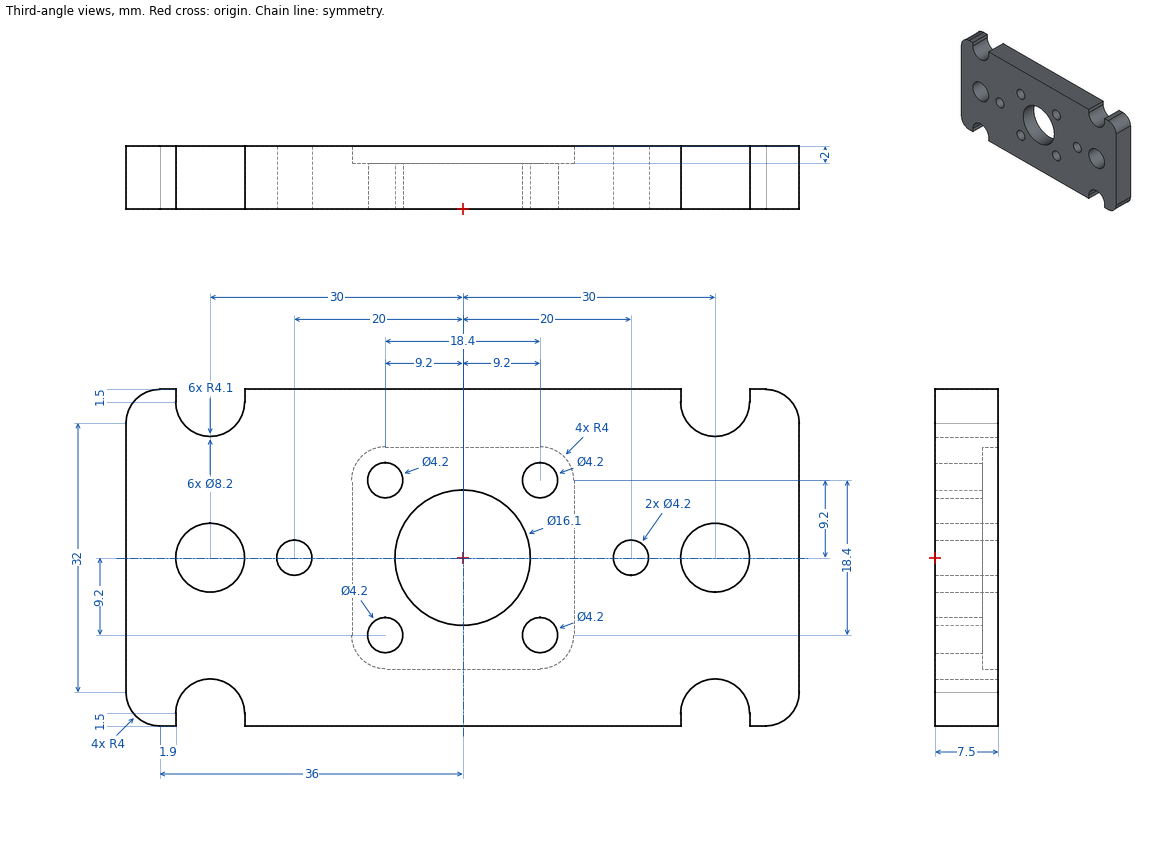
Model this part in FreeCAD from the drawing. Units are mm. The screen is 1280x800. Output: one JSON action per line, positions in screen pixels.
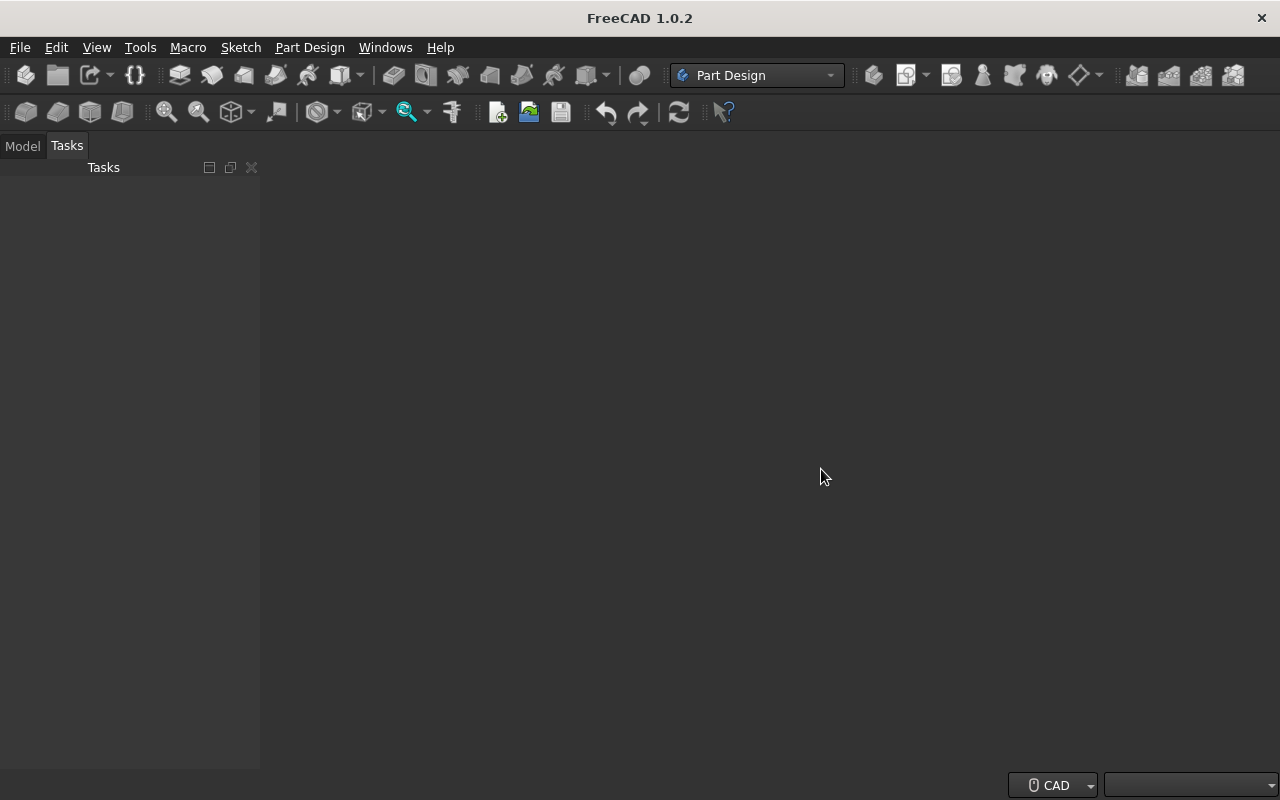
{"action": "left_click", "coordinate": [498, 112]}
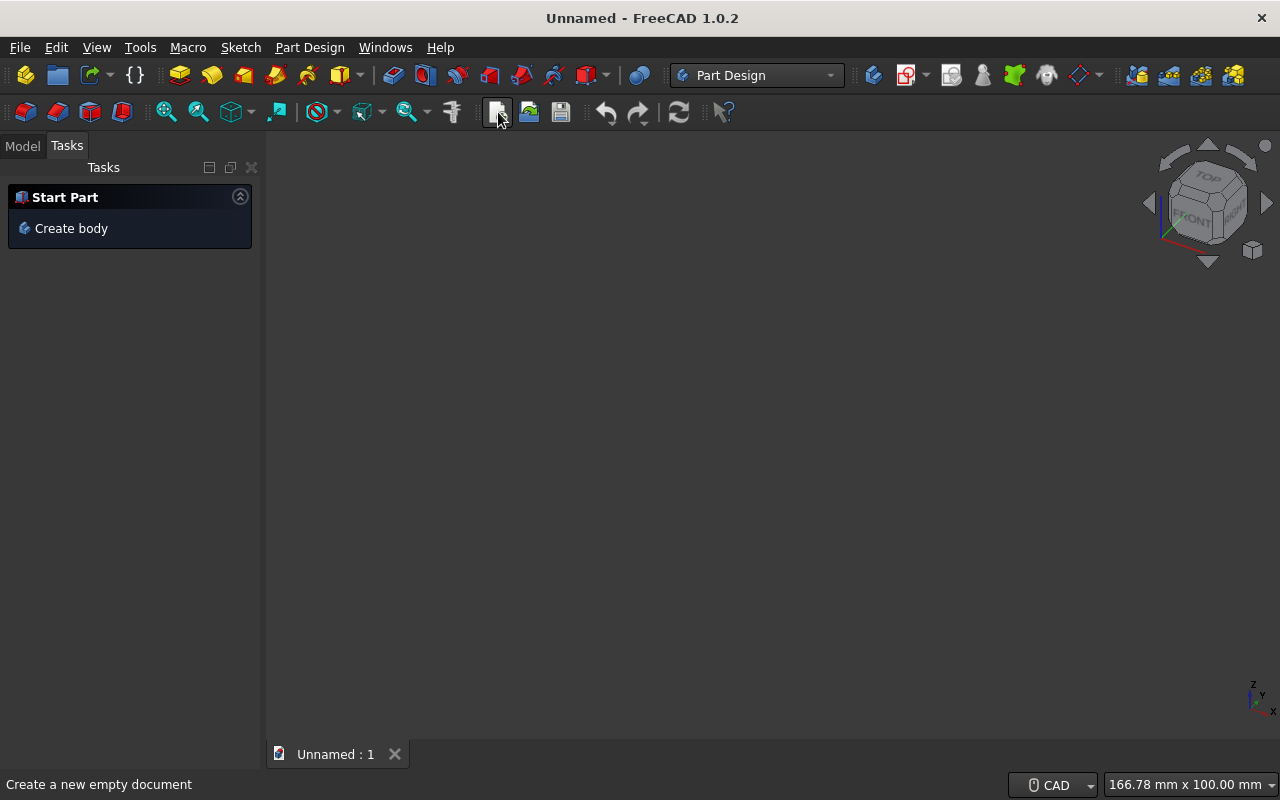
{"action": "left_click", "coordinate": [906, 76]}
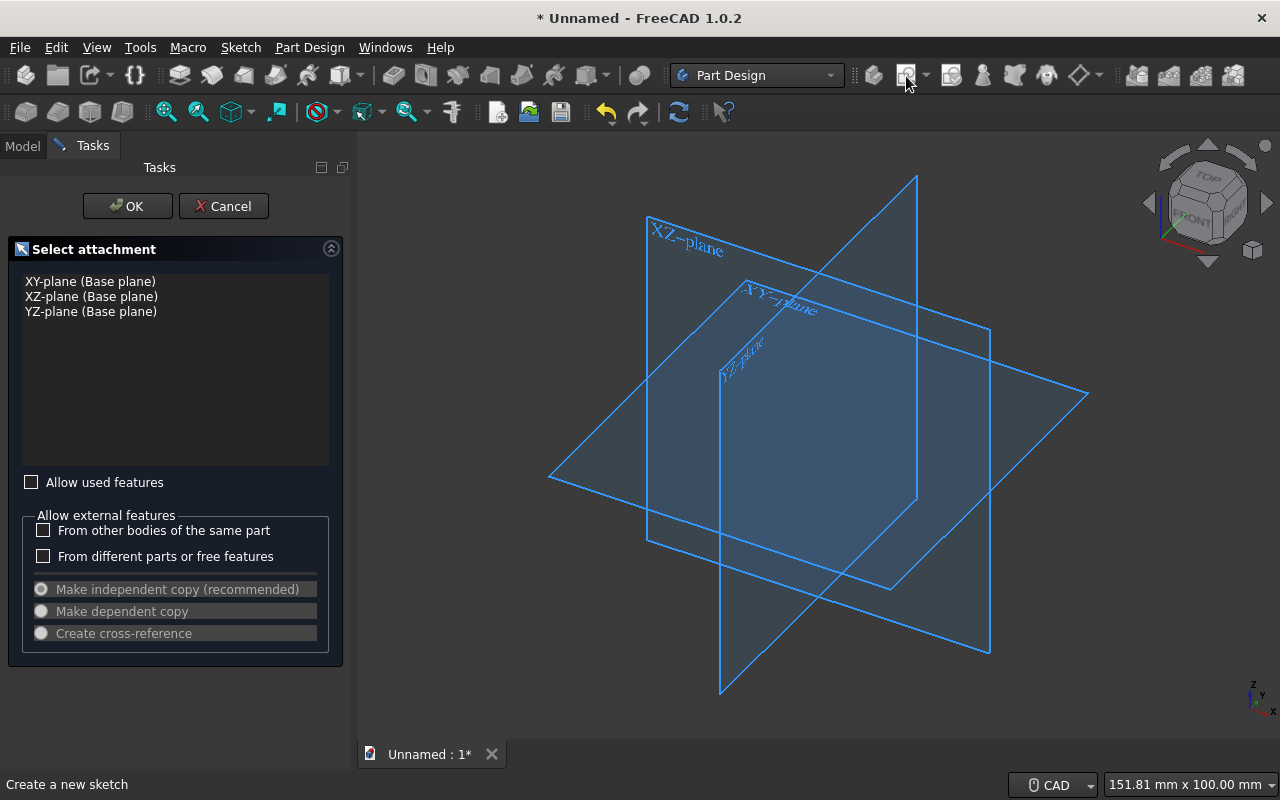
{"action": "left_click", "coordinate": [82, 296]}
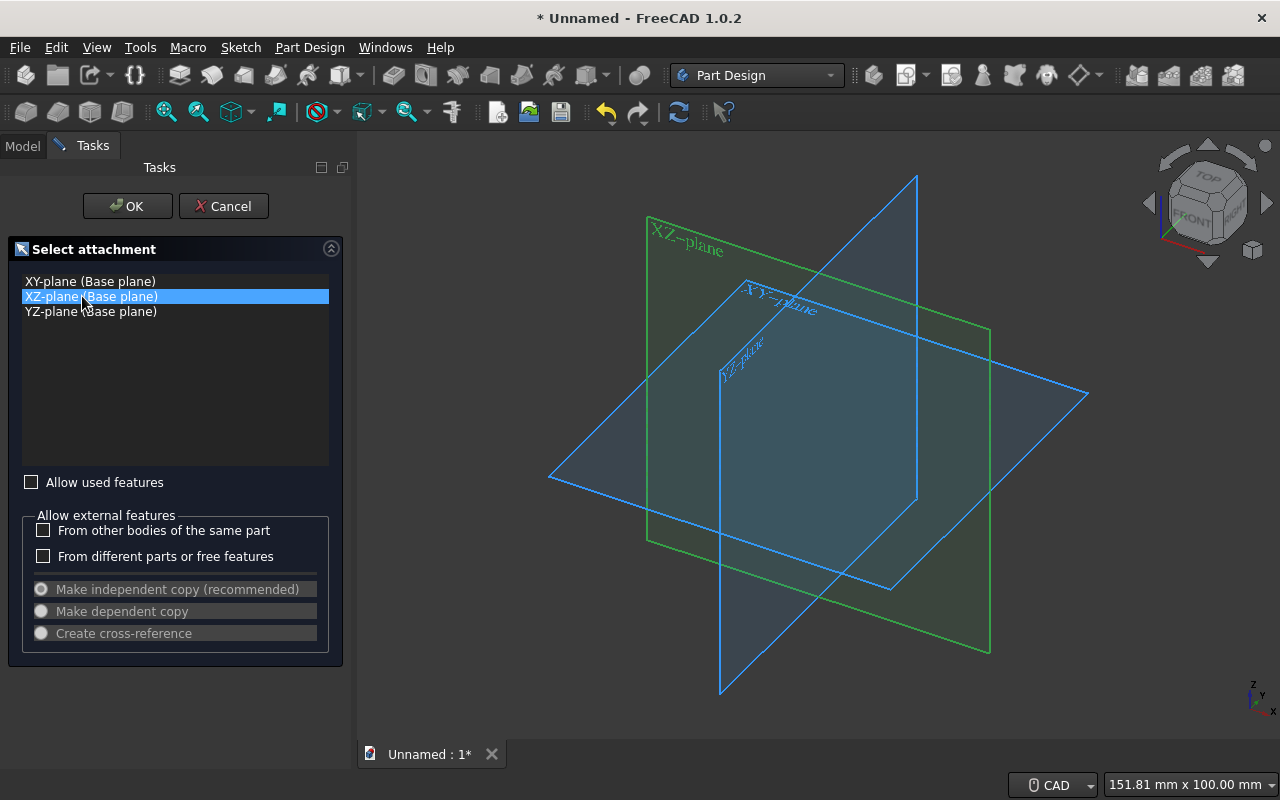
{"action": "left_click", "coordinate": [128, 206]}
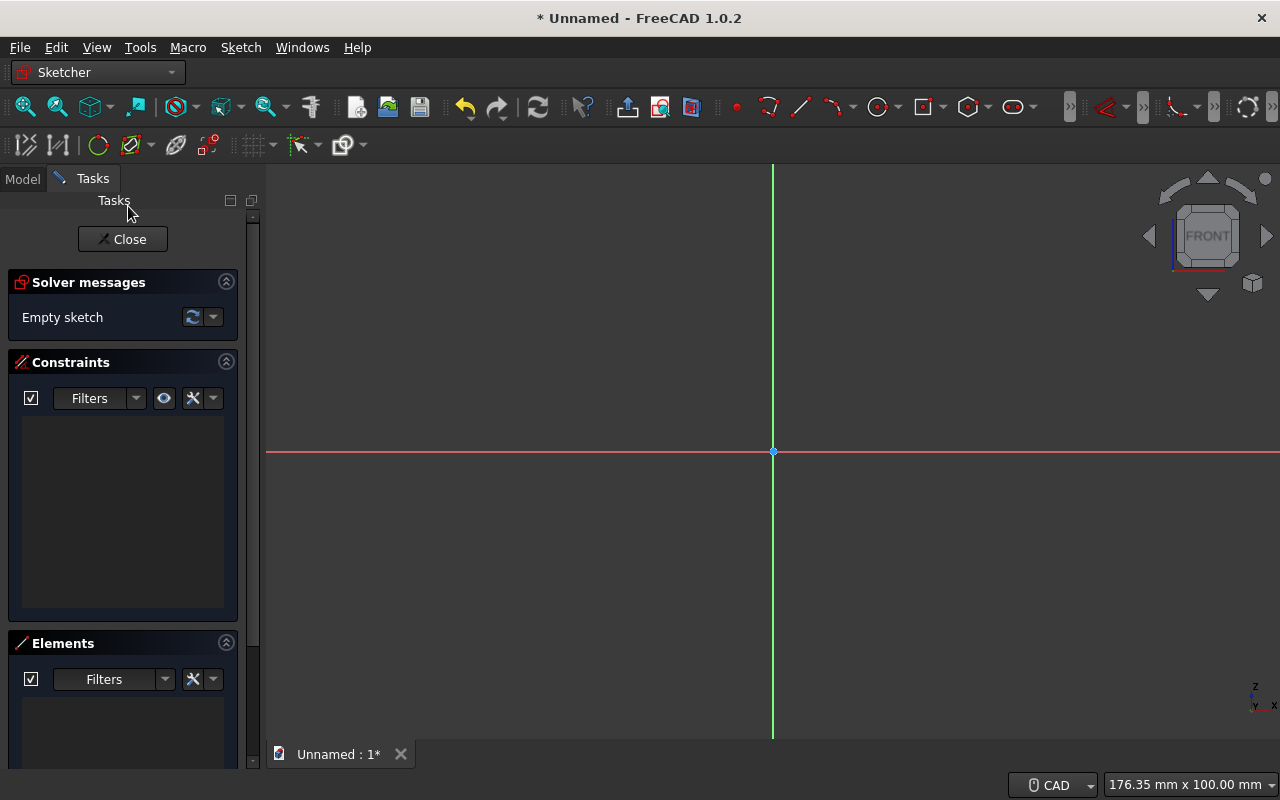
{"action": "left_click", "coordinate": [770, 108]}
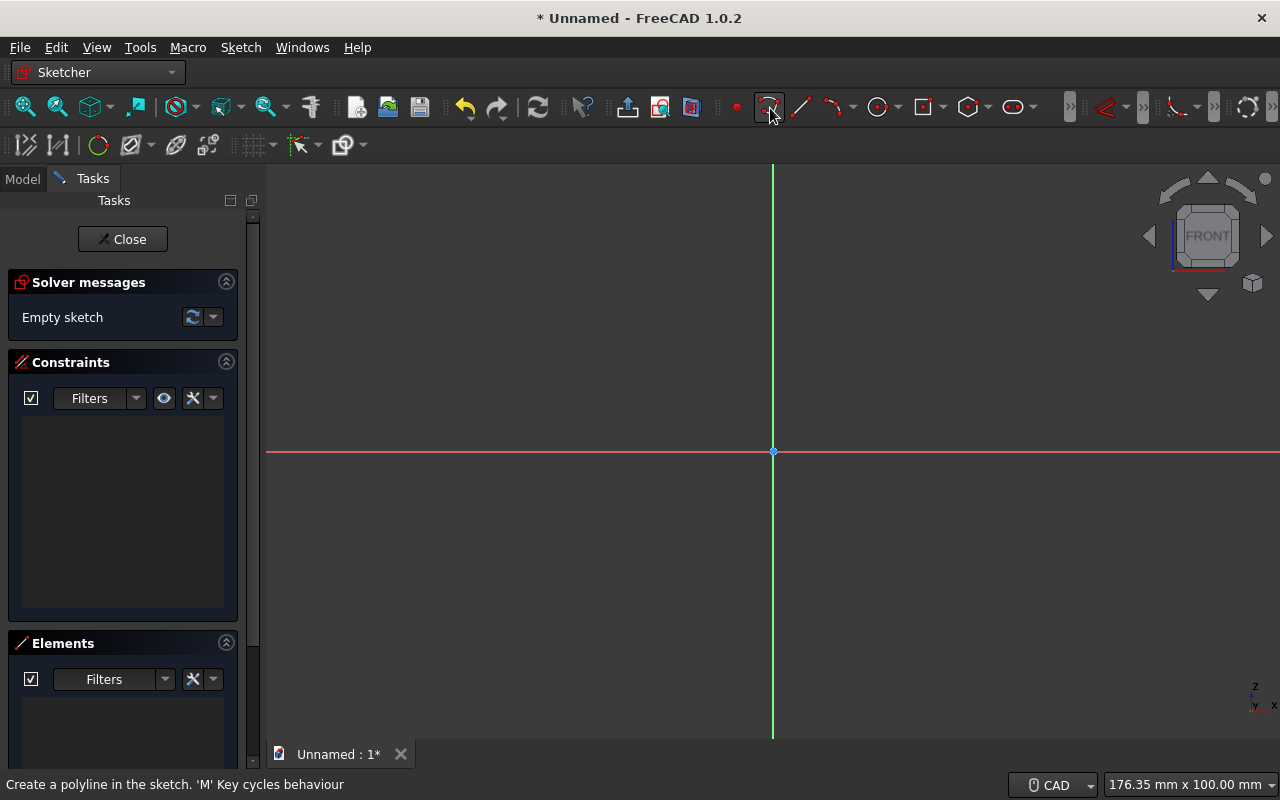
{"action": "left_click", "coordinate": [577, 558]}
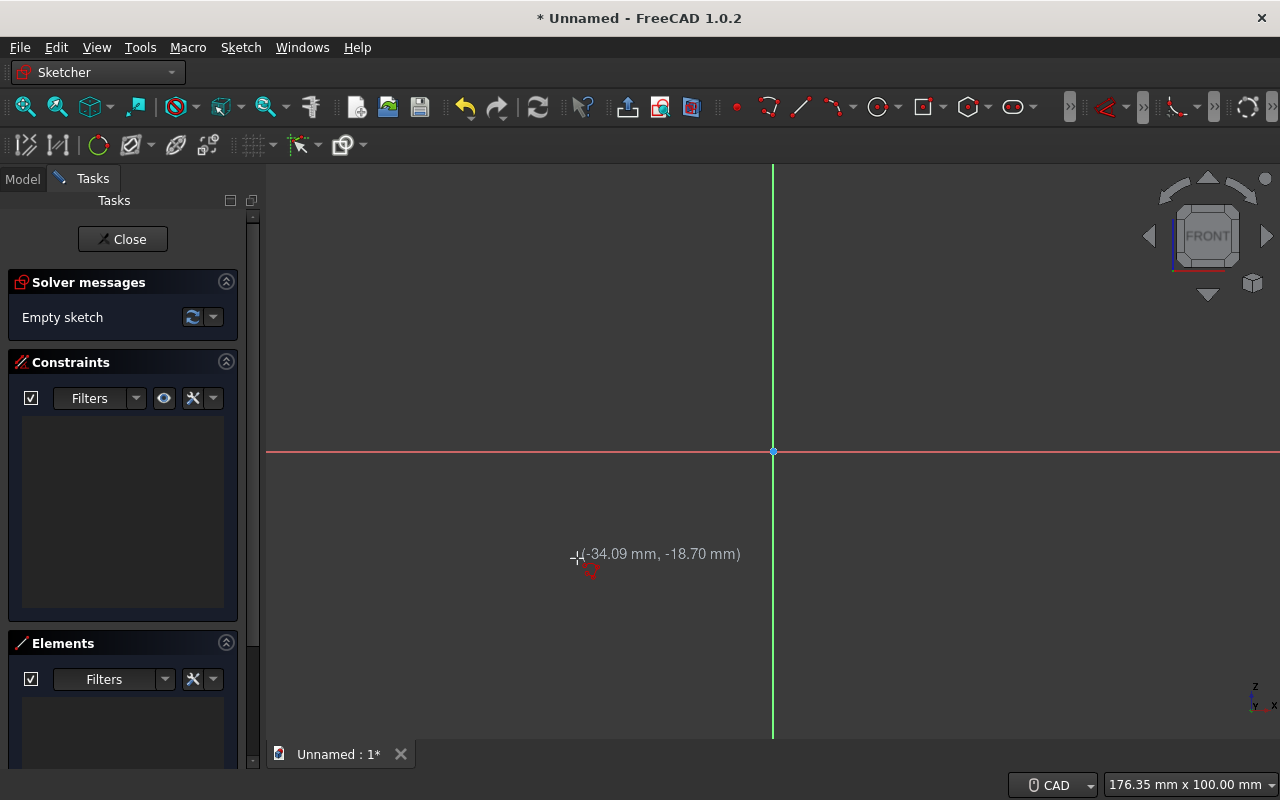
{"action": "scroll", "coordinate": [577, 566], "scroll_direction": "up", "scroll_amount": 4}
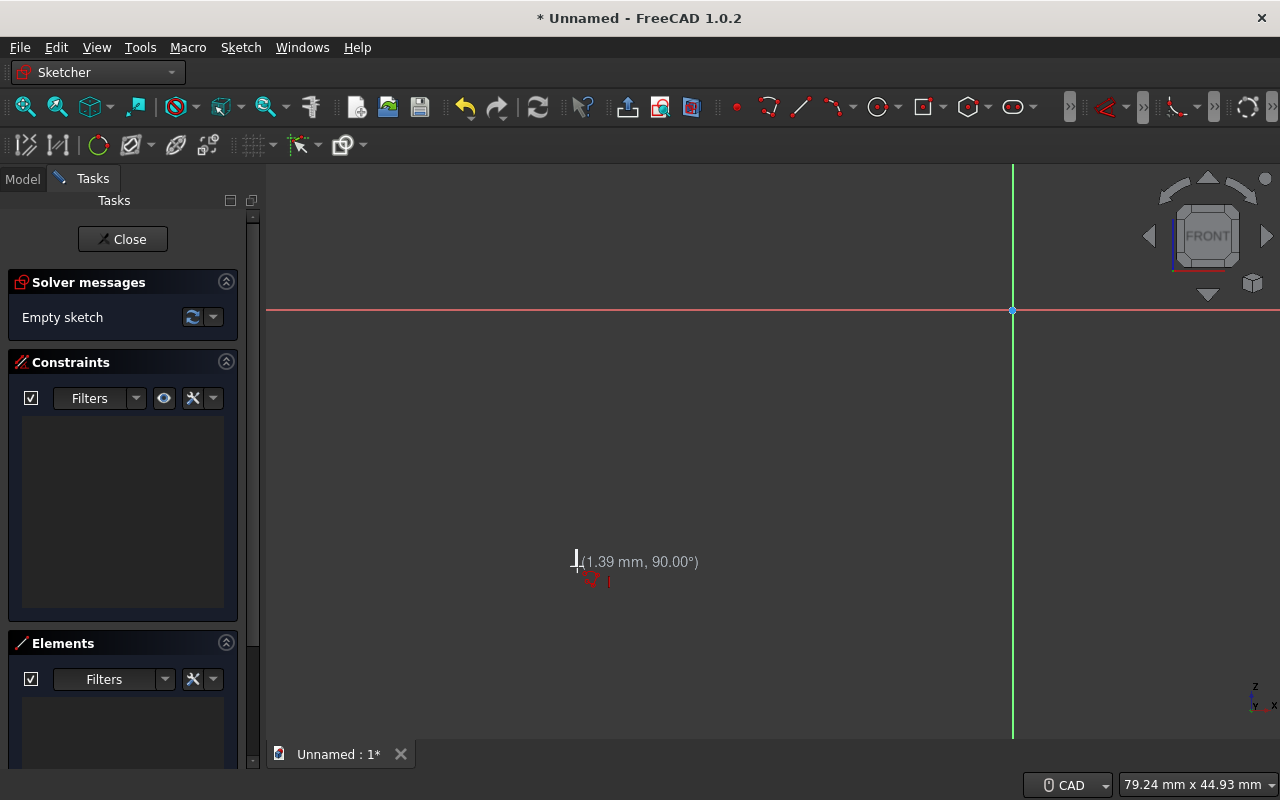
{"action": "left_click", "coordinate": [577, 566]}
{"action": "left_click", "coordinate": [552, 566]}
{"action": "right_click", "coordinate": [552, 566]}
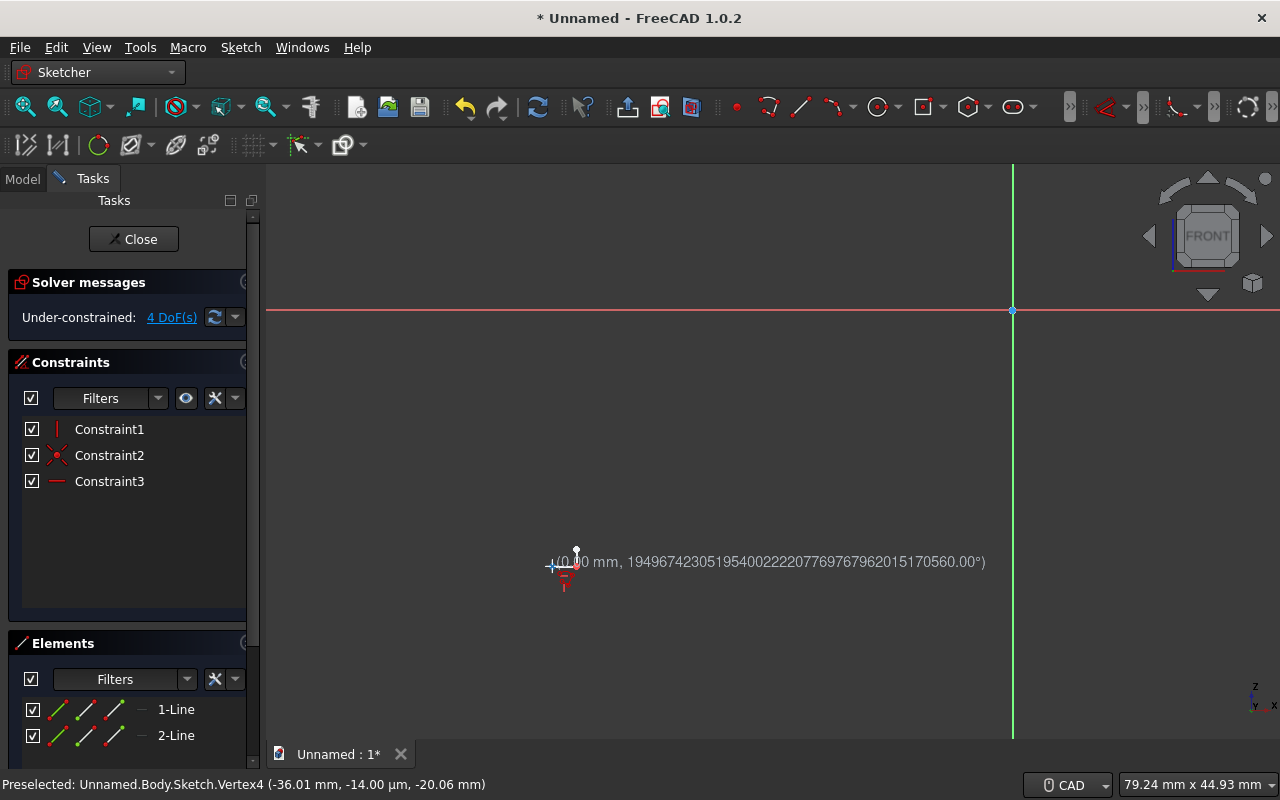
{"action": "left_click", "coordinate": [802, 108]}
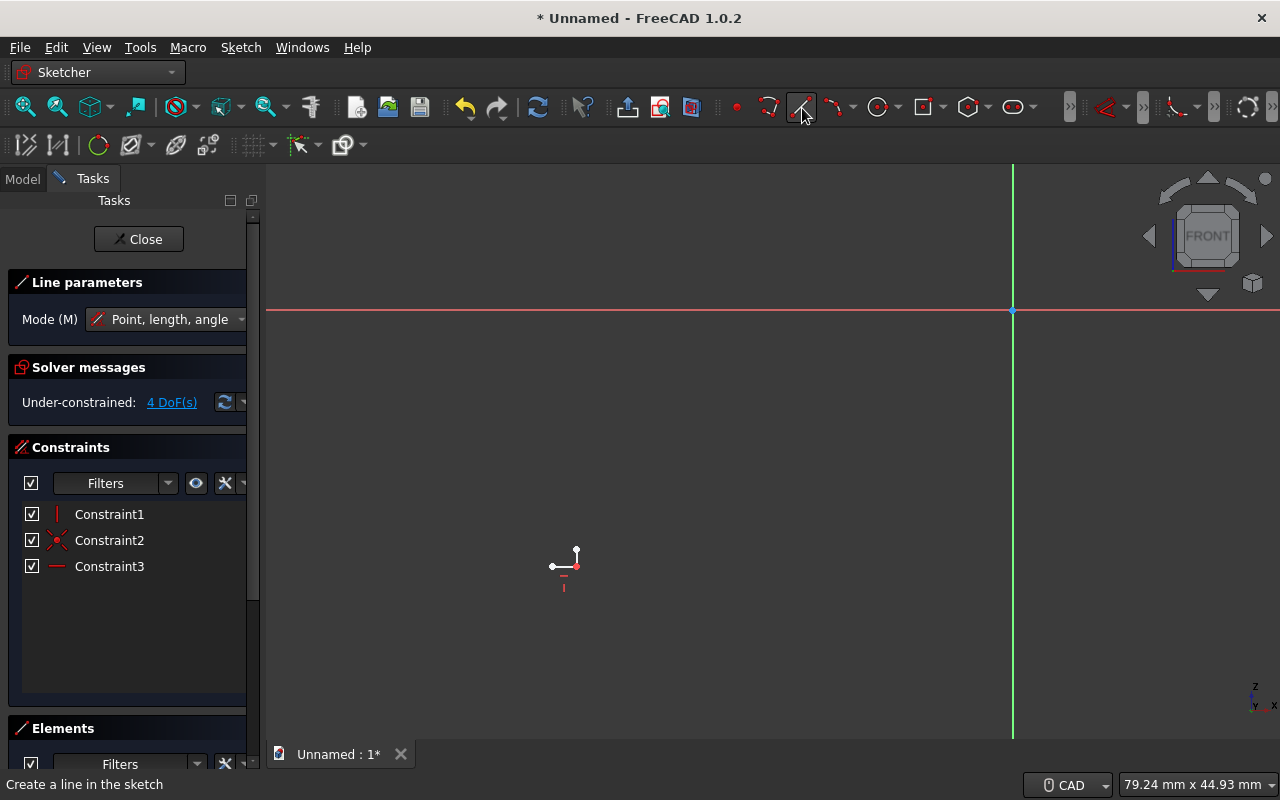
{"action": "left_click", "coordinate": [501, 515]}